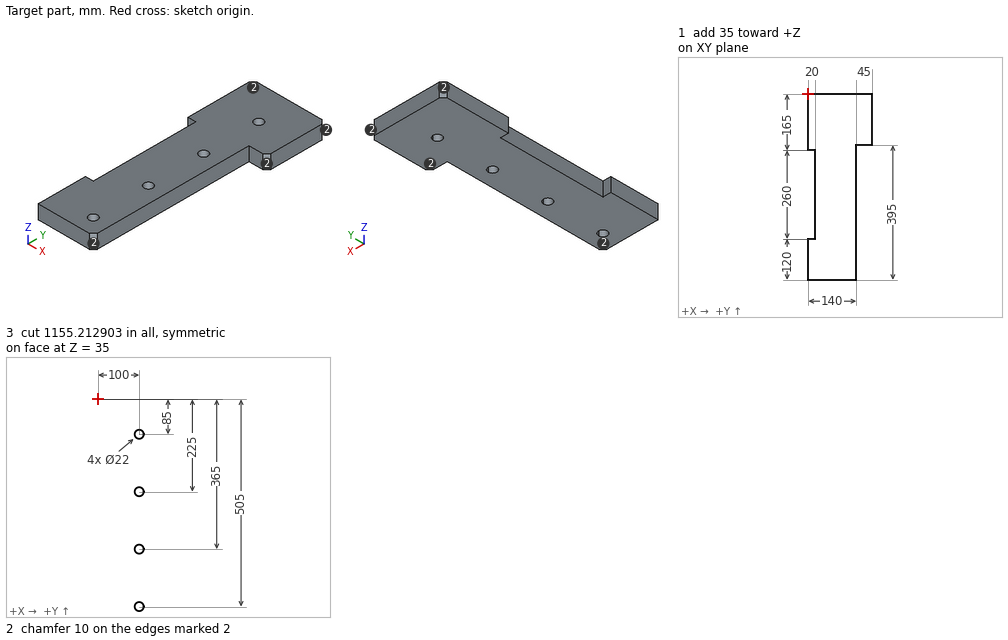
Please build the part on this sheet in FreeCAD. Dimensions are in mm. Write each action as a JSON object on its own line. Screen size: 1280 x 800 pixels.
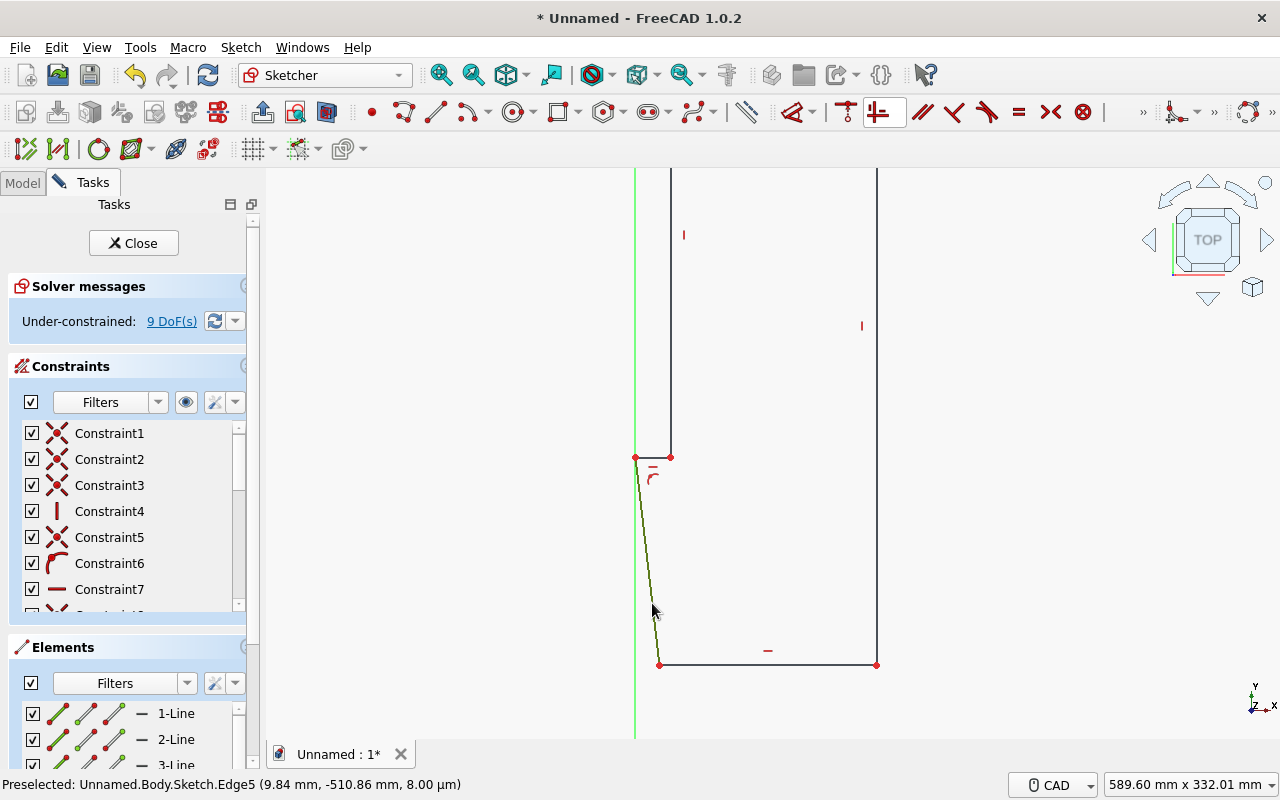
{"action": "left_click", "coordinate": [900, 112]}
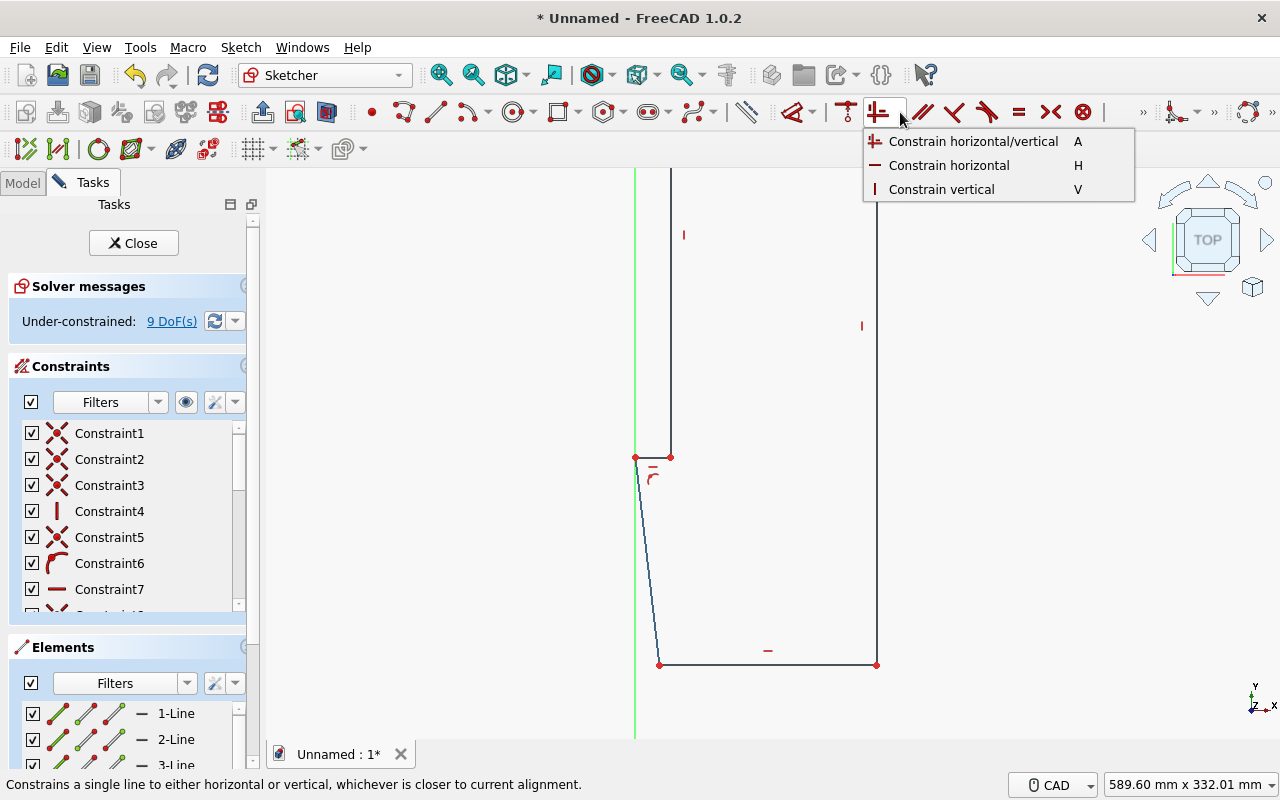
{"action": "left_click", "coordinate": [999, 189]}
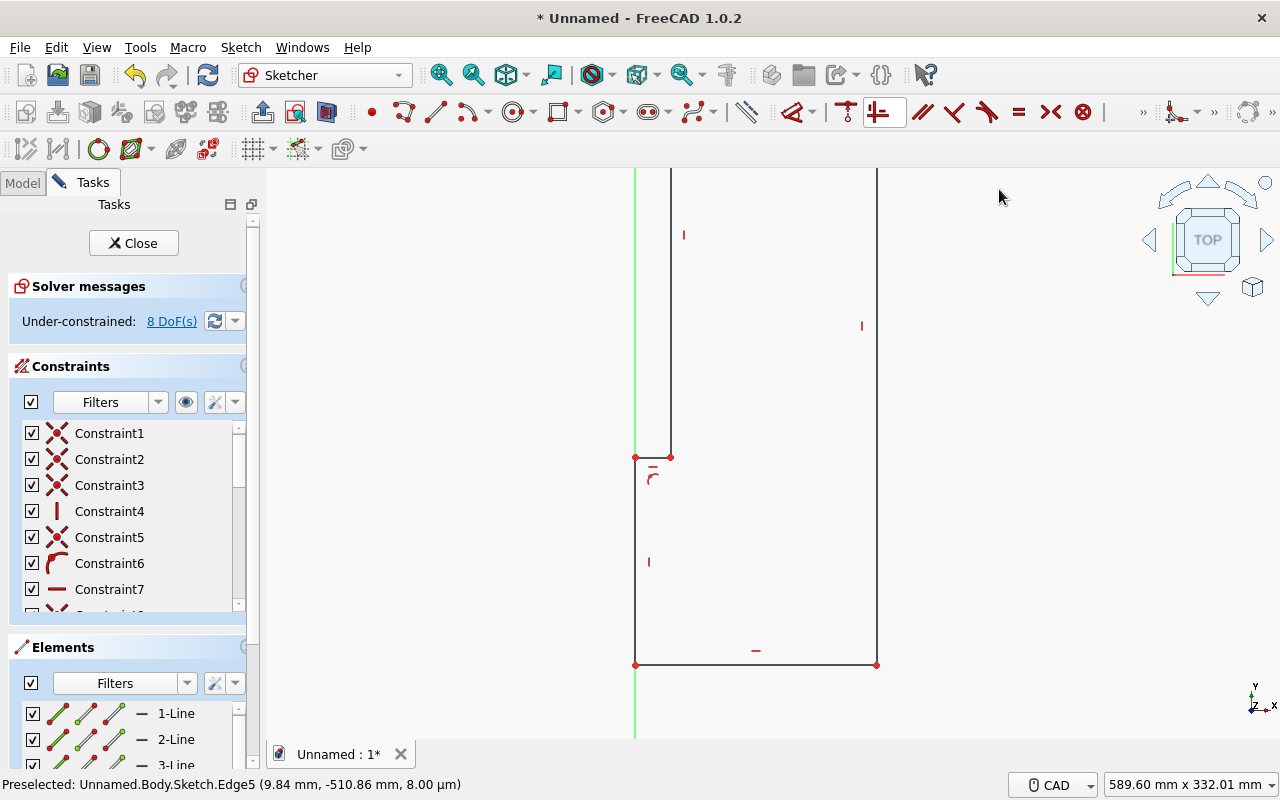
{"action": "scroll", "coordinate": [652, 605], "scroll_direction": "down", "scroll_amount": 5}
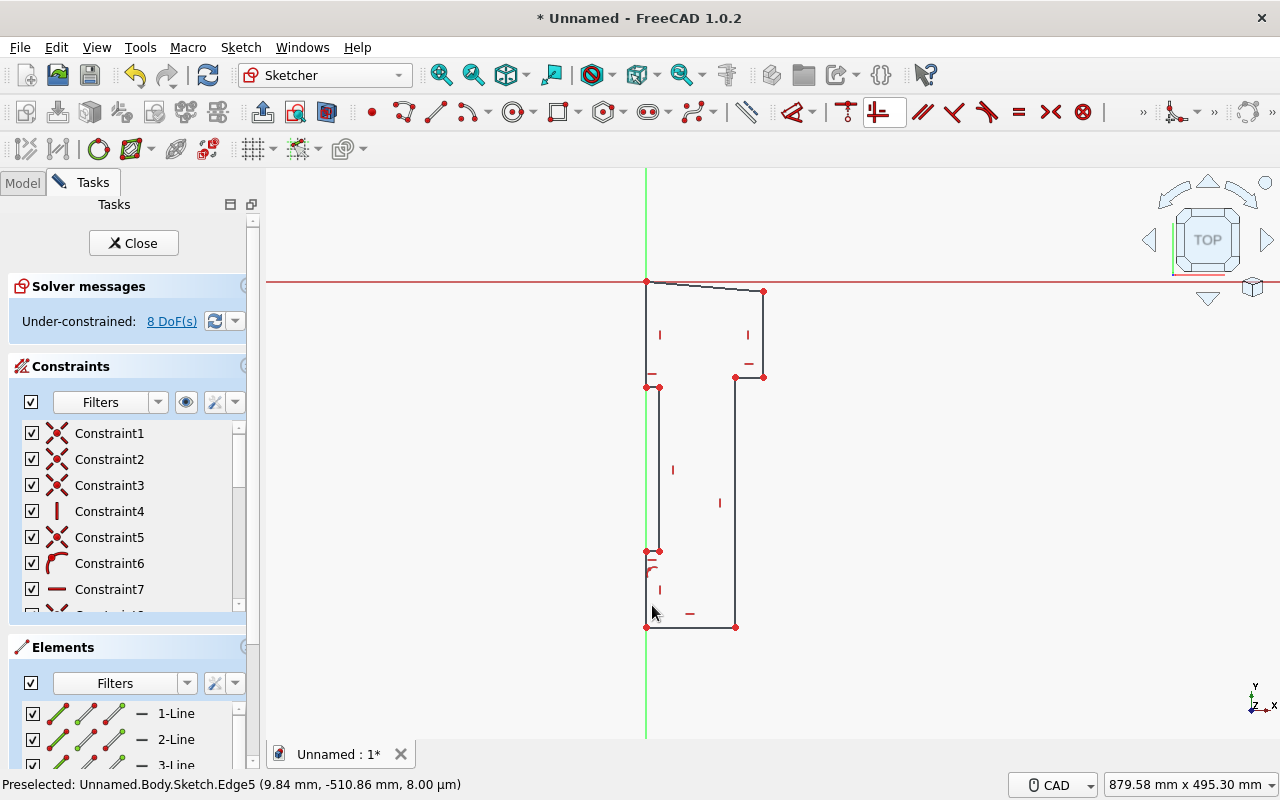
{"action": "scroll", "coordinate": [728, 289], "scroll_direction": "up", "scroll_amount": 4}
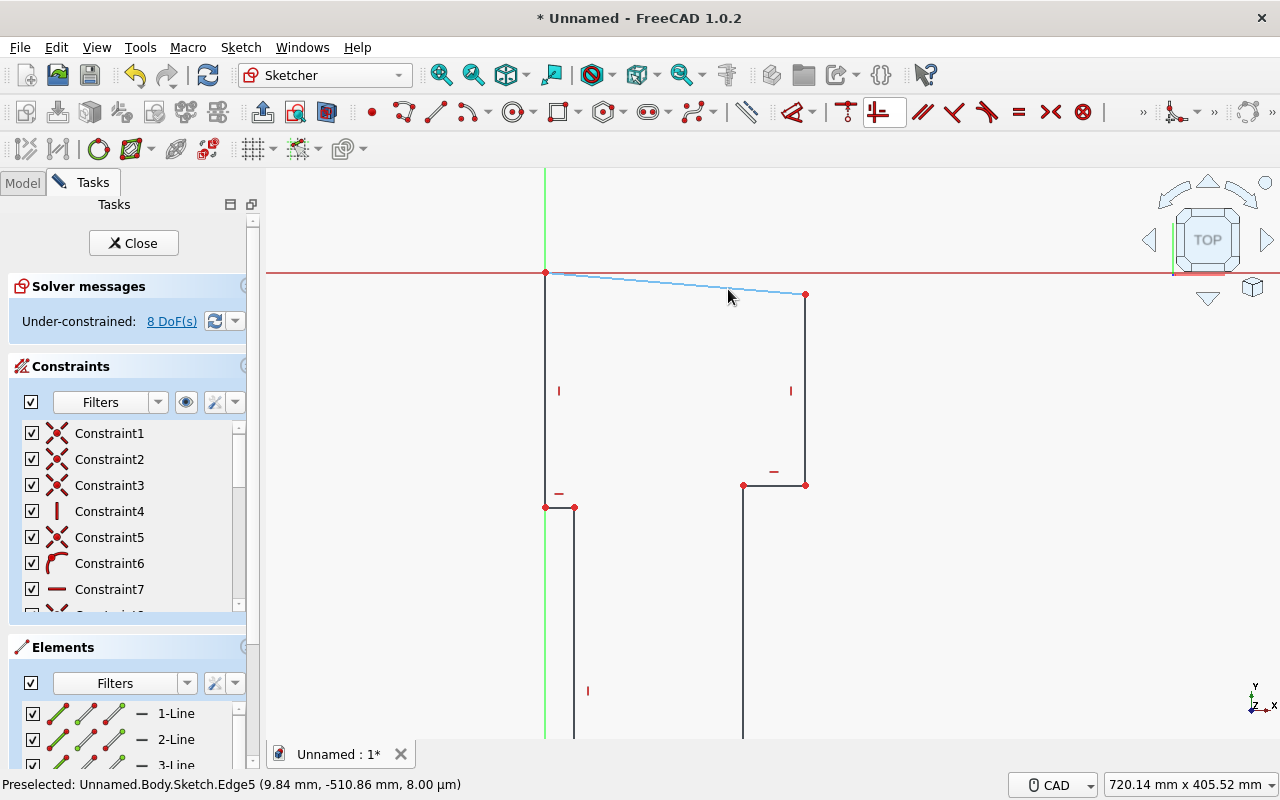
{"action": "left_click", "coordinate": [727, 288]}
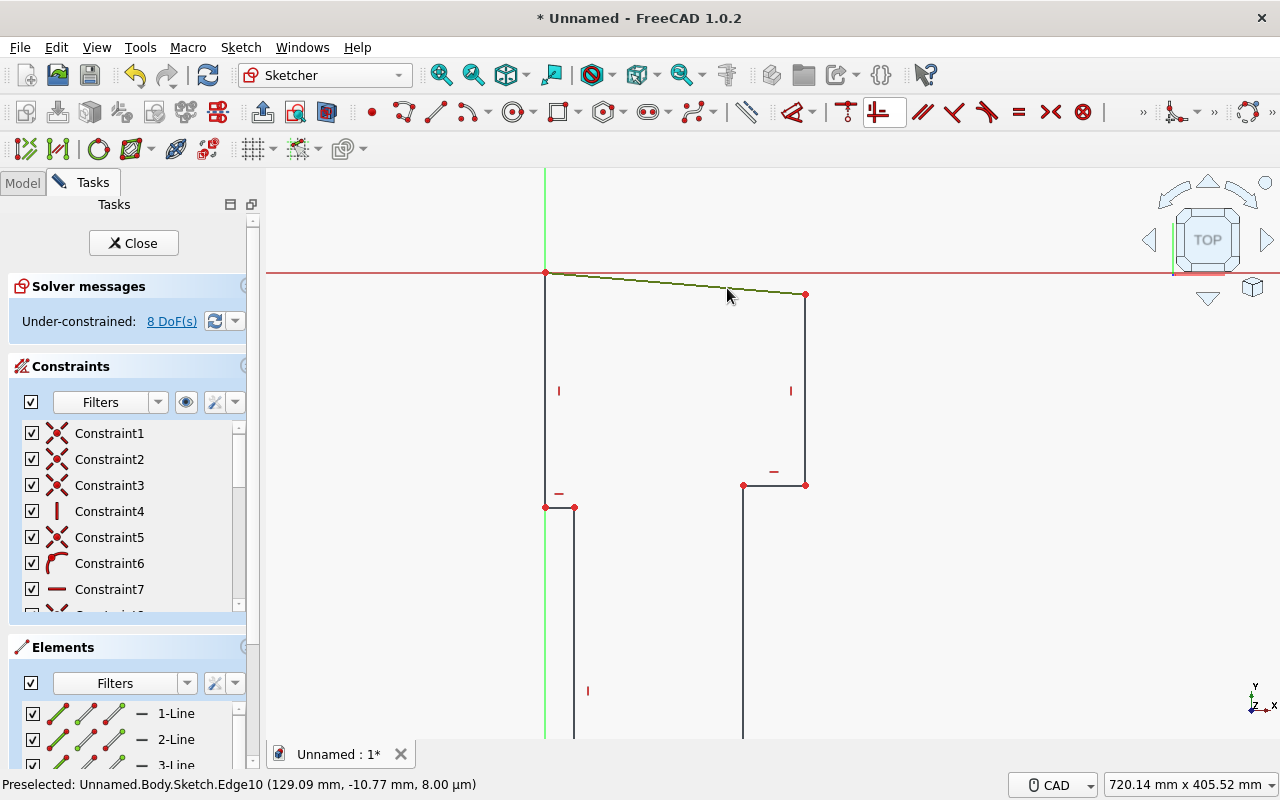
{"action": "key", "text": "h"}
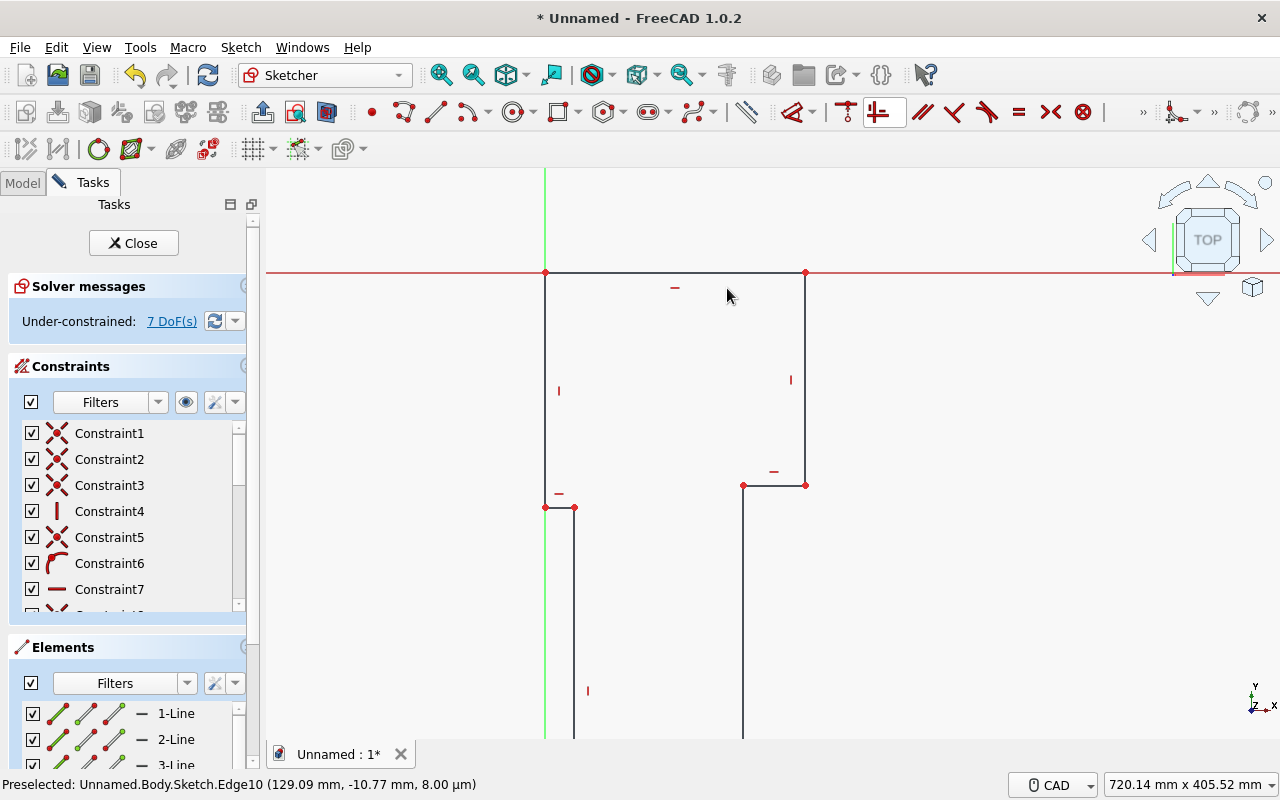
{"action": "left_click", "coordinate": [792, 112]}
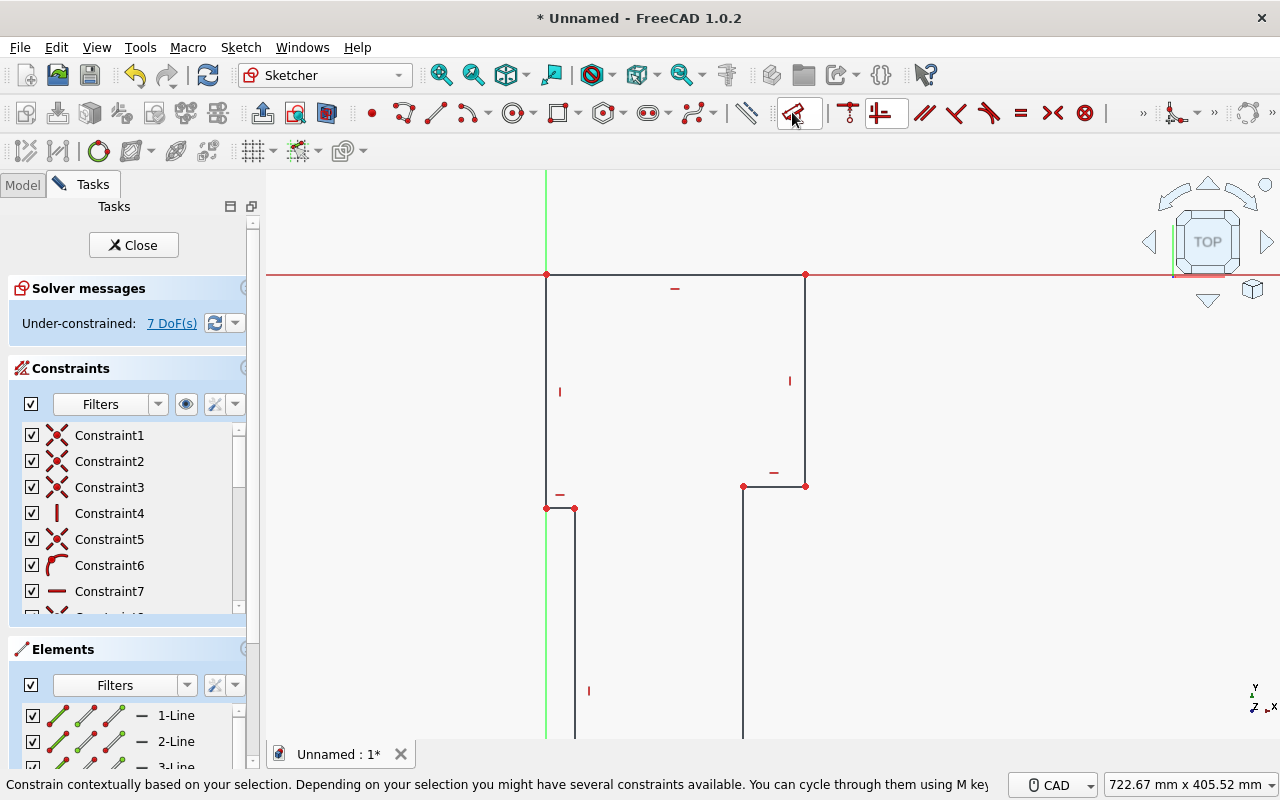
{"action": "scroll", "coordinate": [558, 508], "scroll_direction": "up", "scroll_amount": 2}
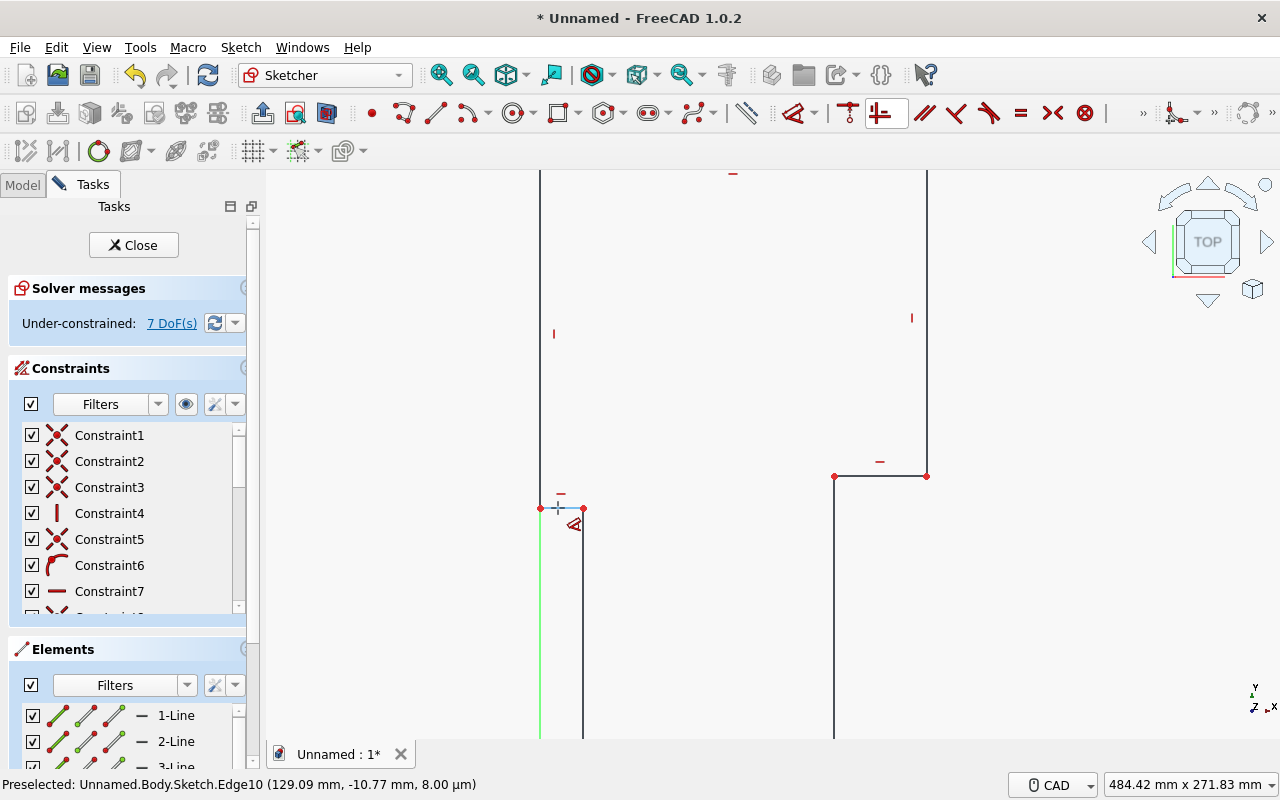
{"action": "left_click", "coordinate": [557, 508]}
{"action": "left_click", "coordinate": [562, 474]}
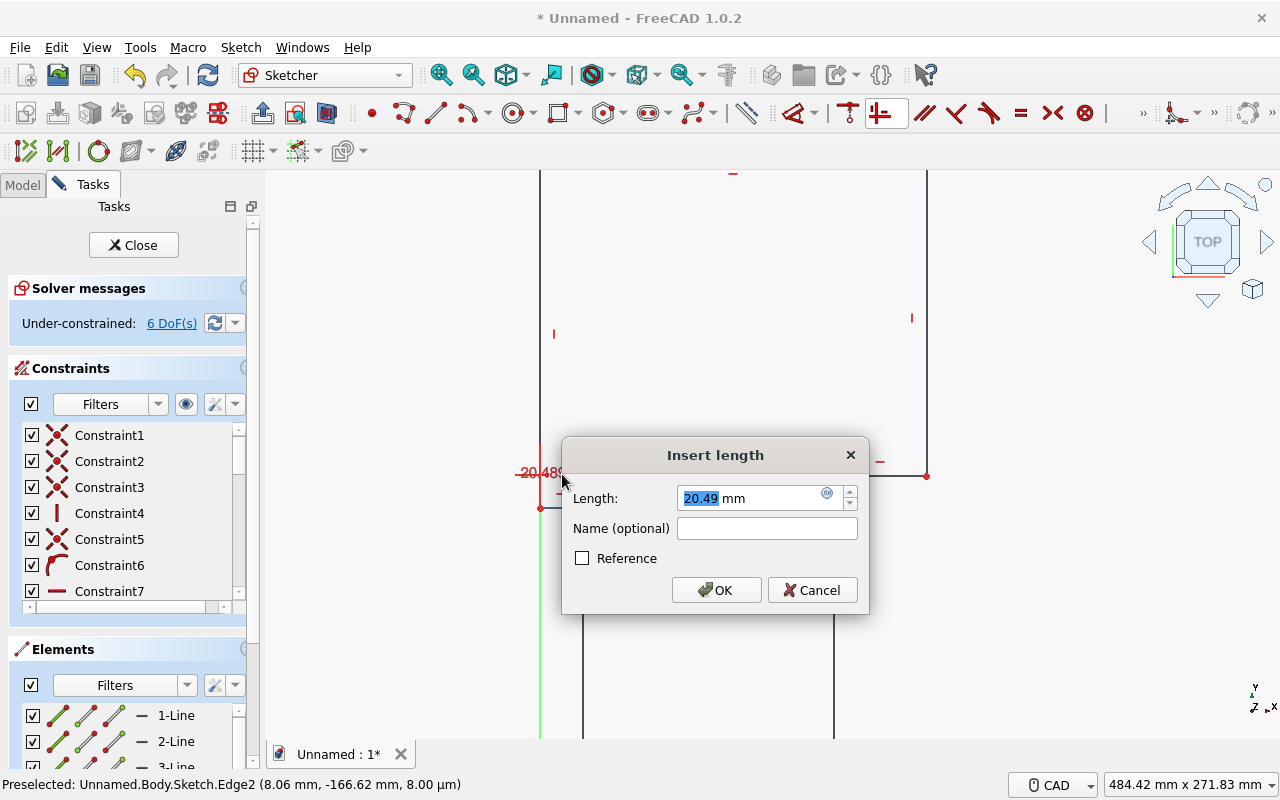
{"action": "type", "text": "20"}
{"action": "key", "text": "Return"}